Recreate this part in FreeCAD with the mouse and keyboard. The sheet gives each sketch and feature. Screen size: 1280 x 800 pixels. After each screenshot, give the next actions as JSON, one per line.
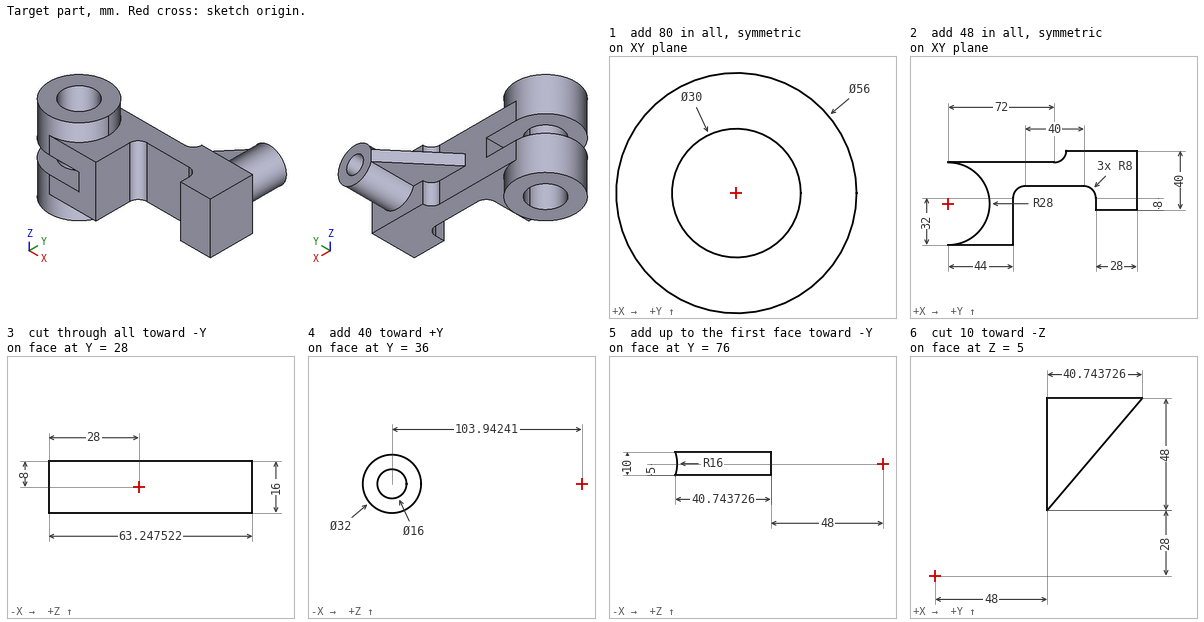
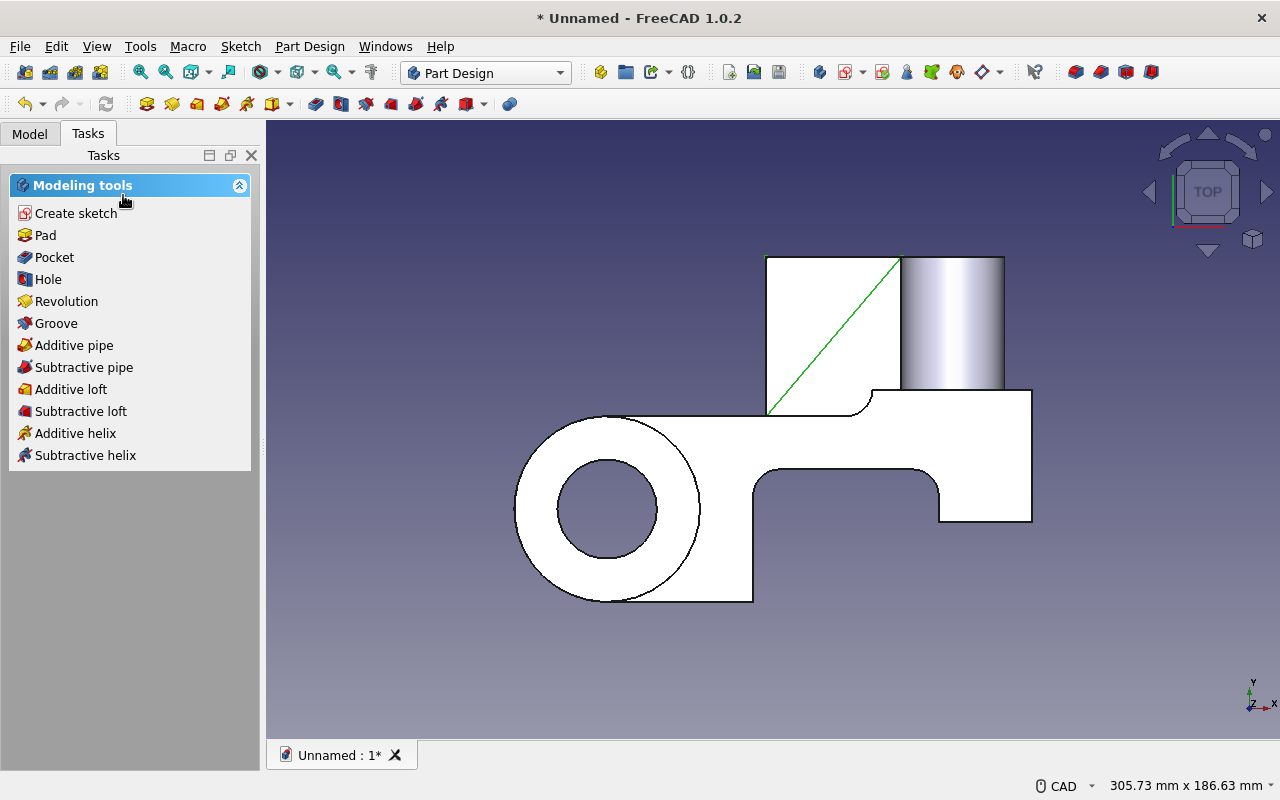
{"action": "left_click", "coordinate": [316, 104]}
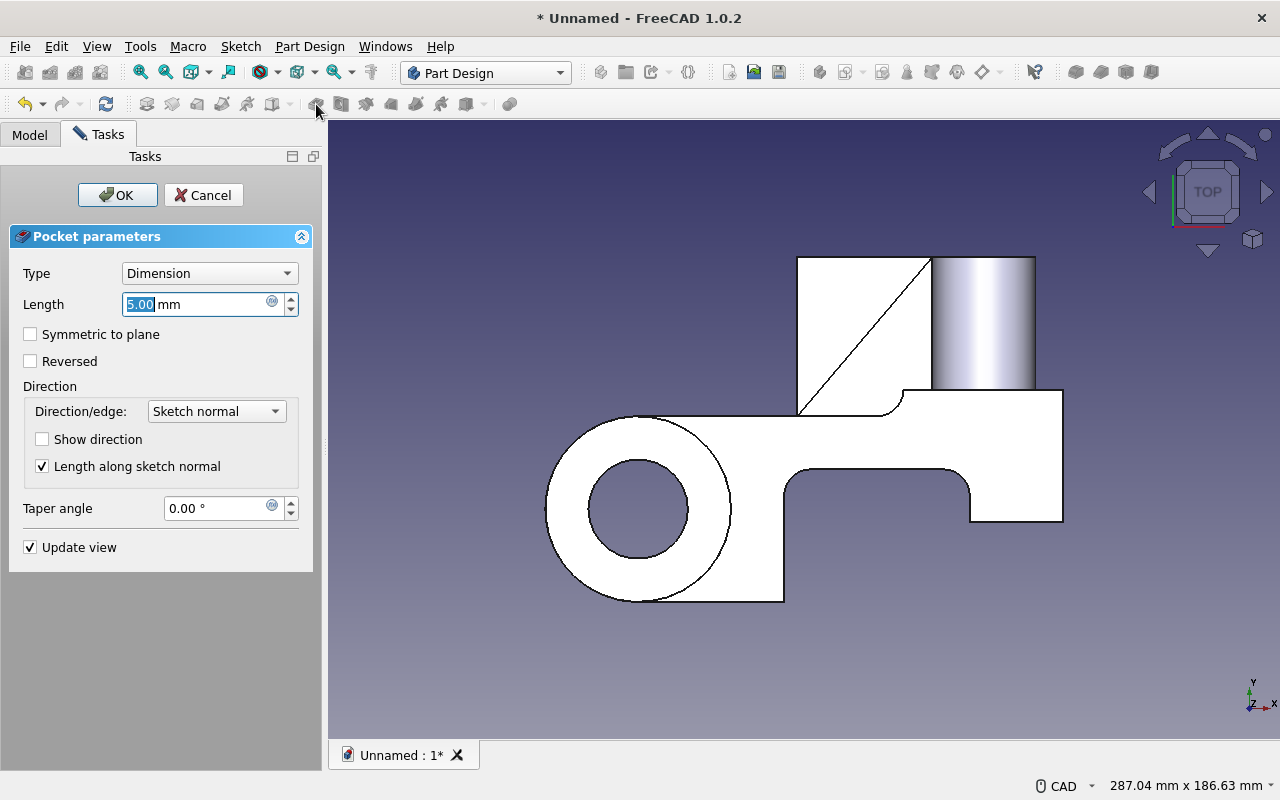
{"action": "type", "text": "10"}
{"action": "key", "text": "Tab"}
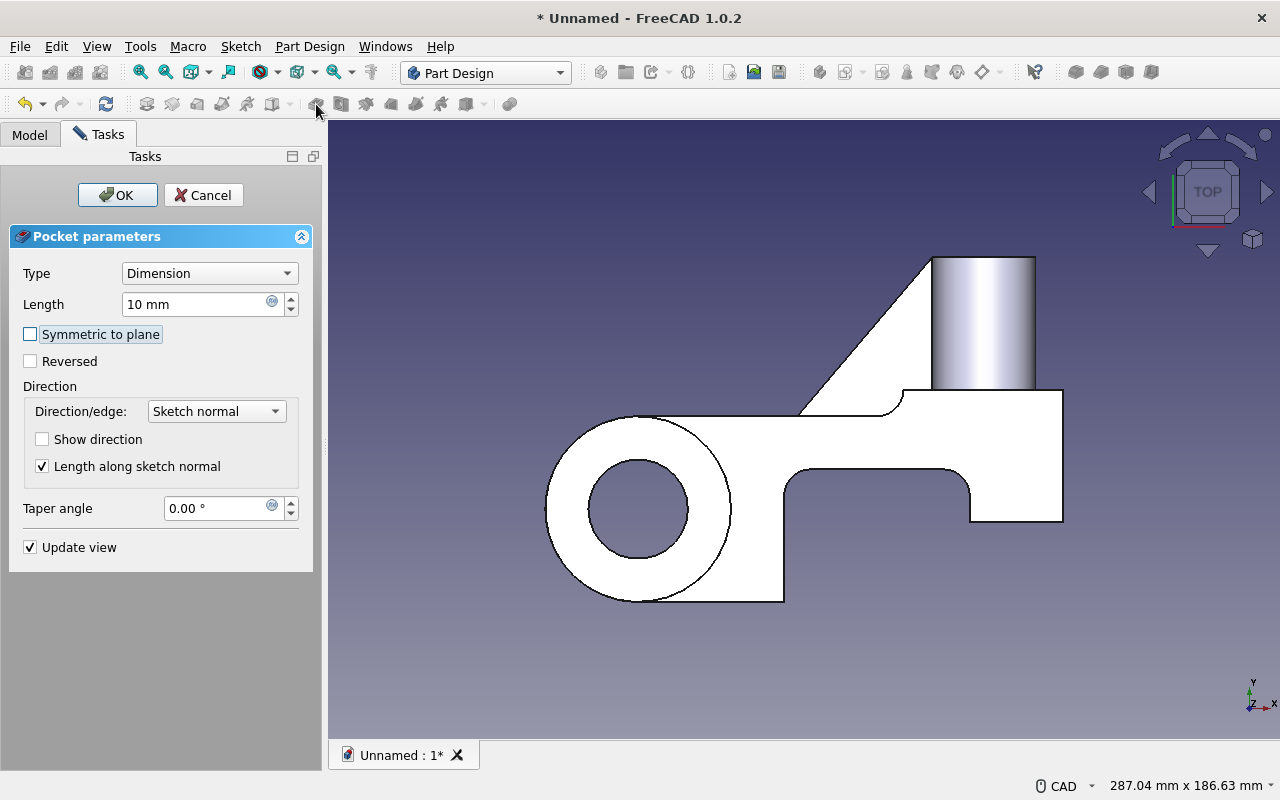
{"action": "left_click", "coordinate": [118, 195]}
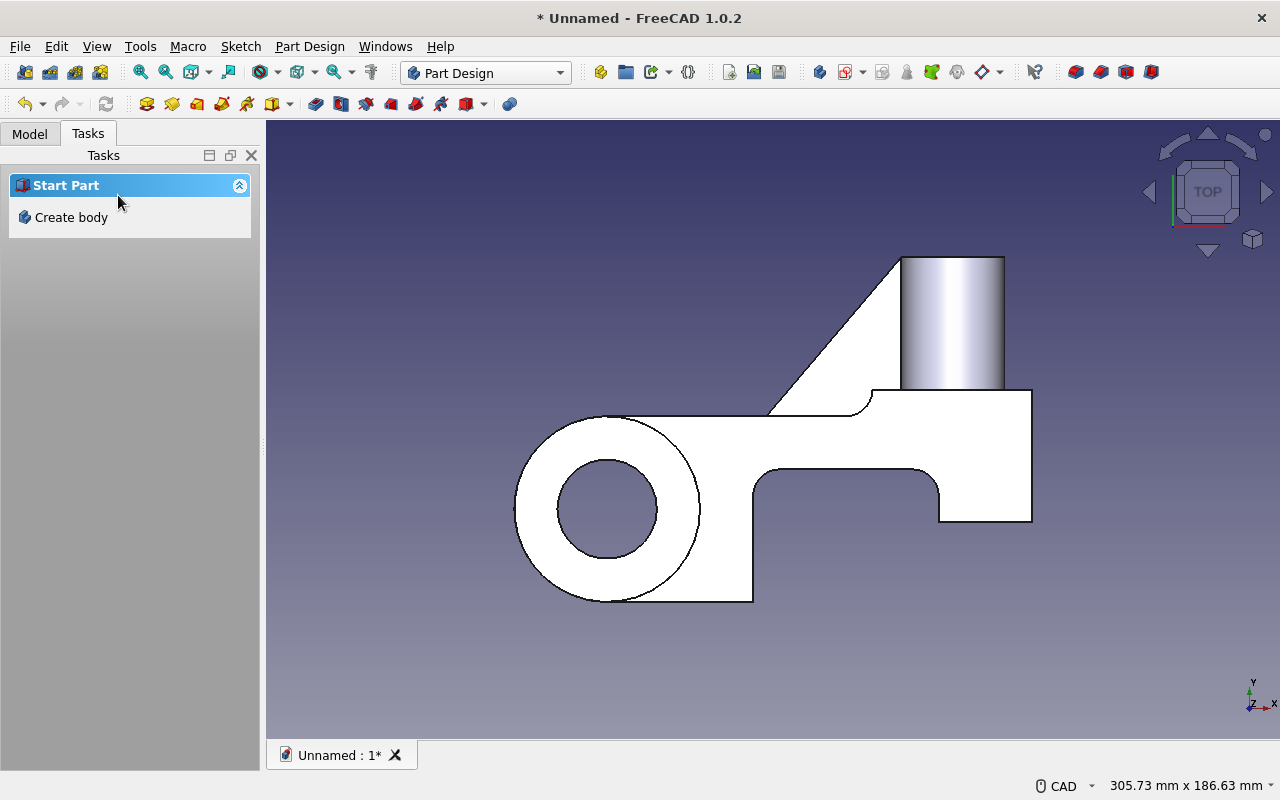
{"action": "key", "text": "0"}